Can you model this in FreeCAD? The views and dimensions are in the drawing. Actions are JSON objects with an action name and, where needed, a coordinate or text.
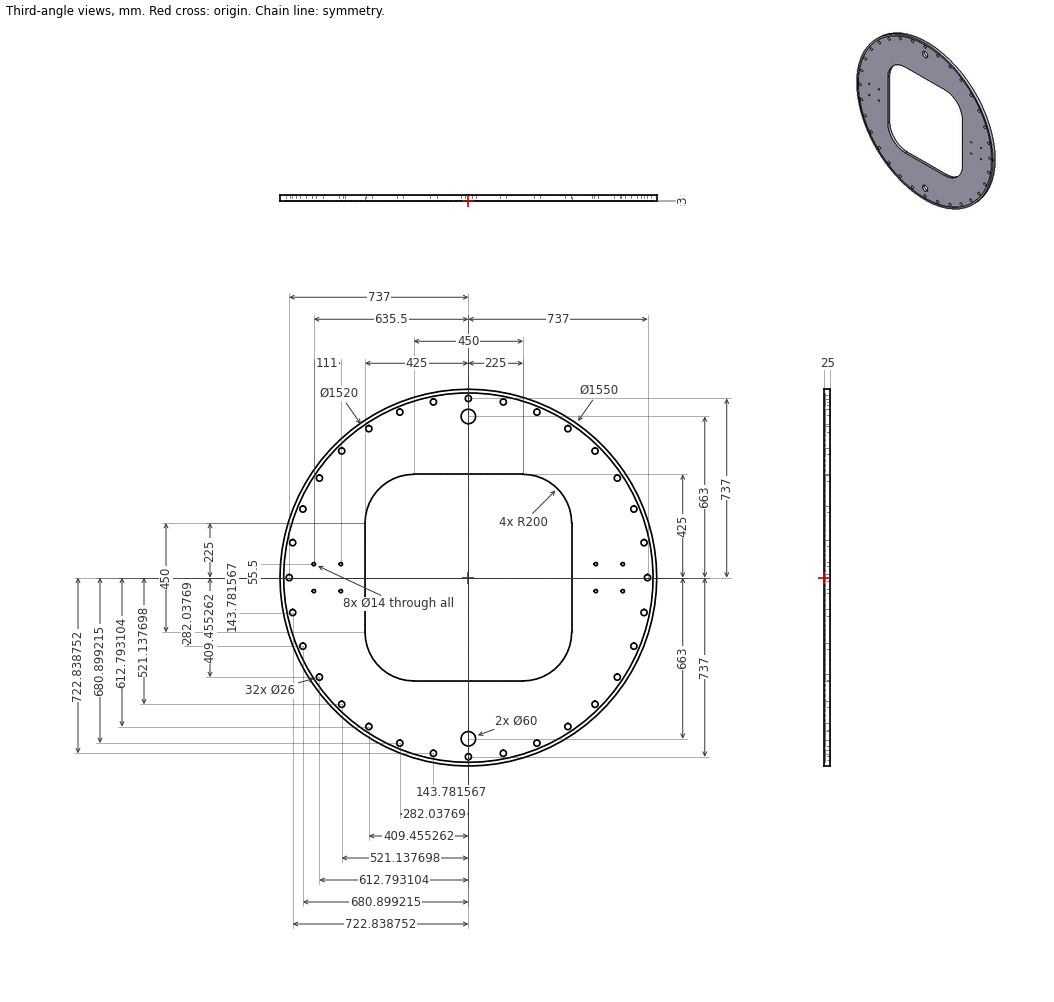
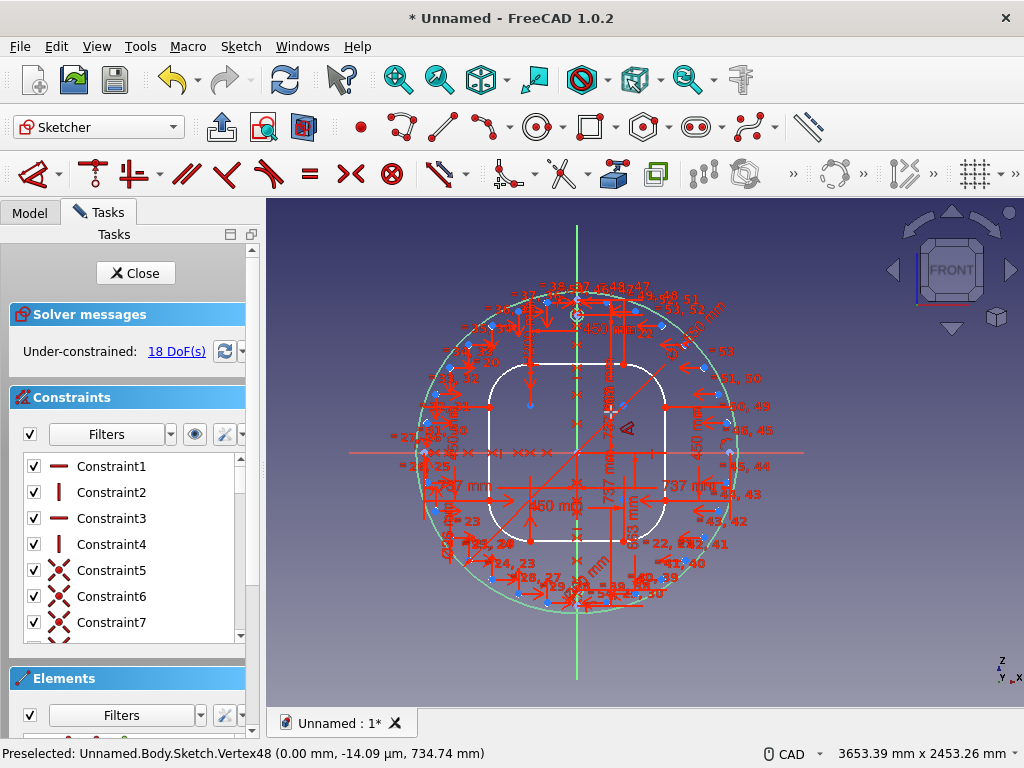
{"action": "left_click", "coordinate": [624, 364]}
{"action": "left_click", "coordinate": [617, 282]}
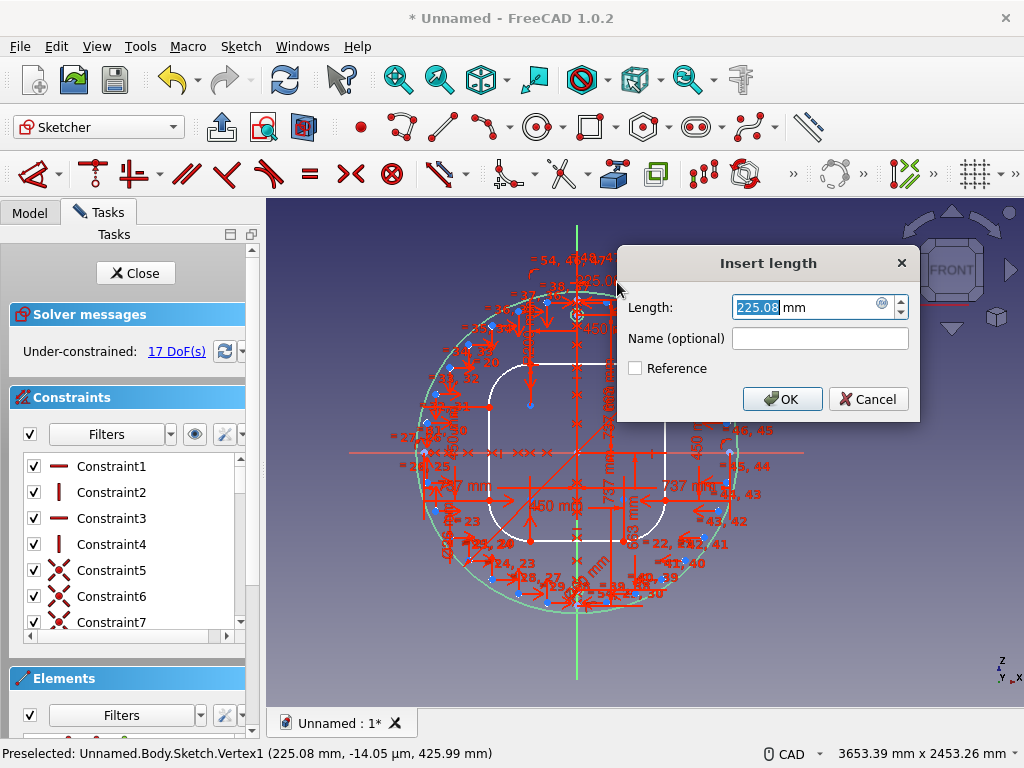
{"action": "type", "text": "225"}
{"action": "key", "text": "Return"}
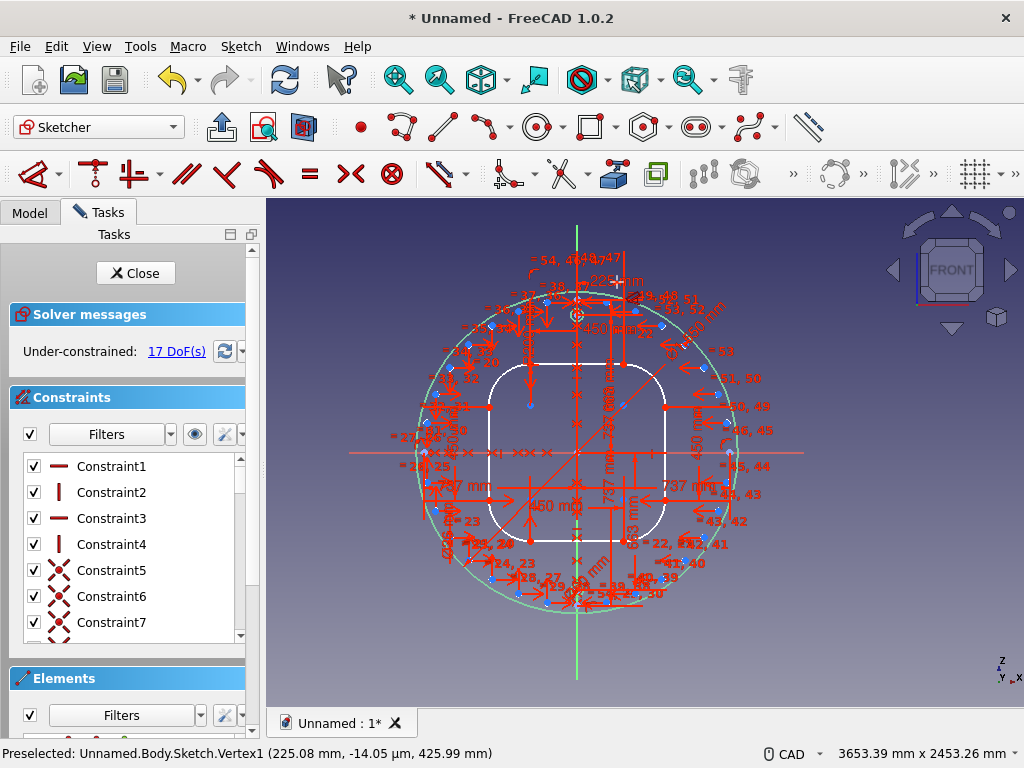
{"action": "left_click", "coordinate": [624, 364]}
{"action": "left_click", "coordinate": [543, 439]}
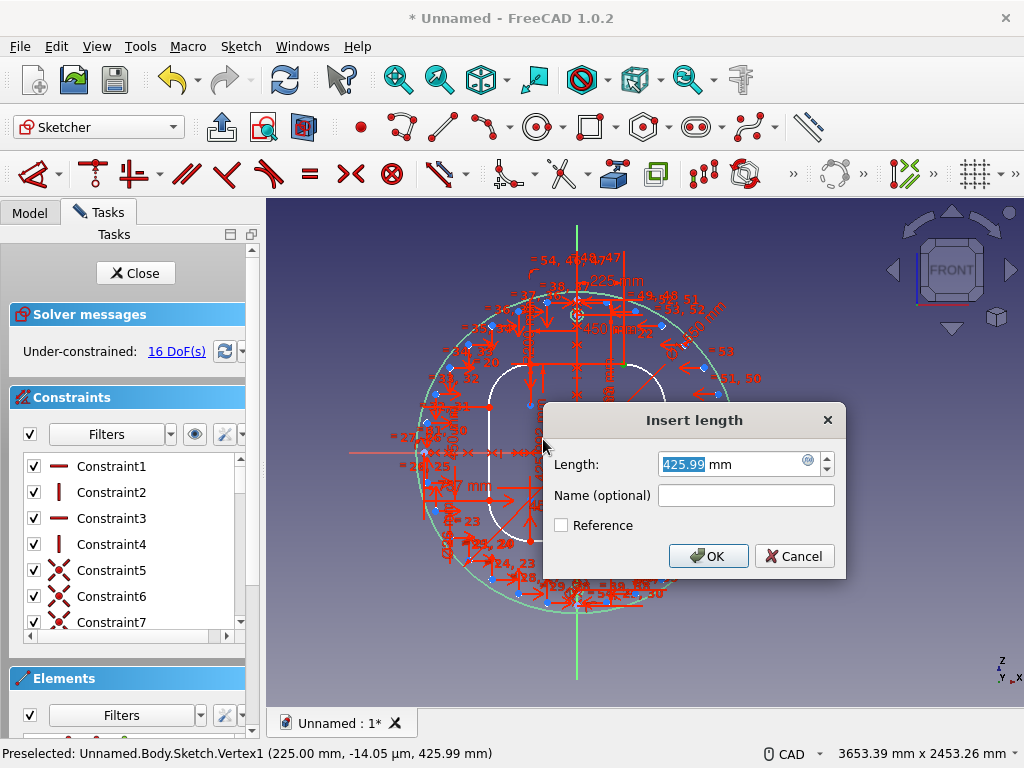
{"action": "type", "text": "425"}
{"action": "key", "text": "Return"}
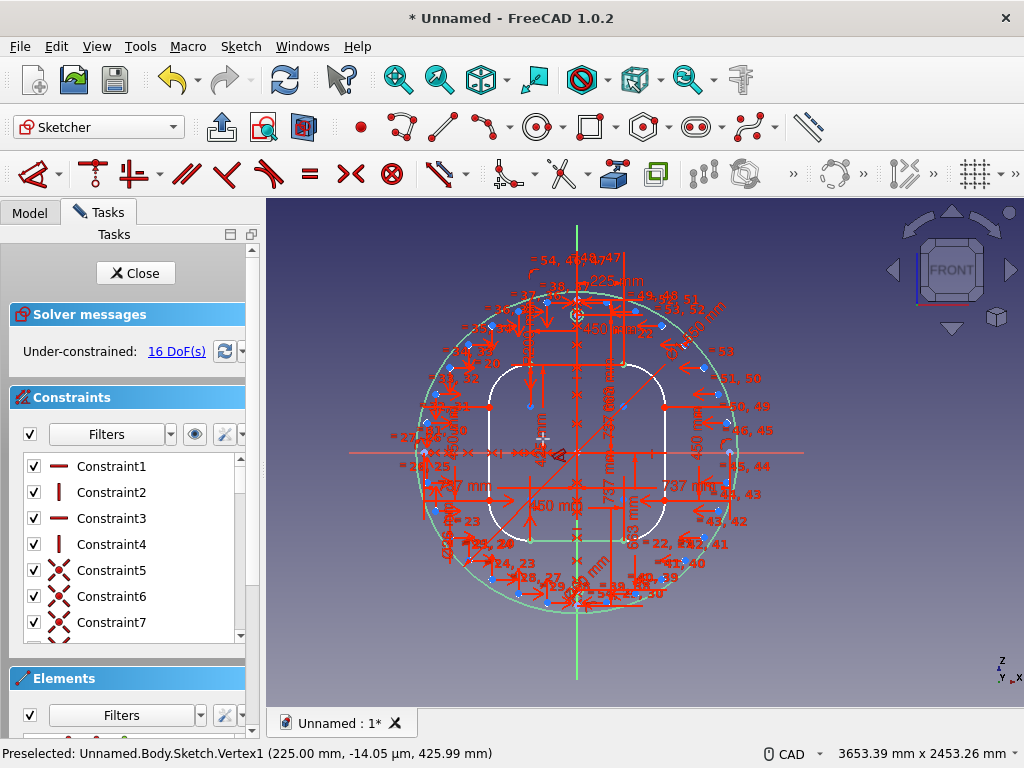
{"action": "left_click", "coordinate": [489, 407]}
{"action": "left_click", "coordinate": [533, 559]}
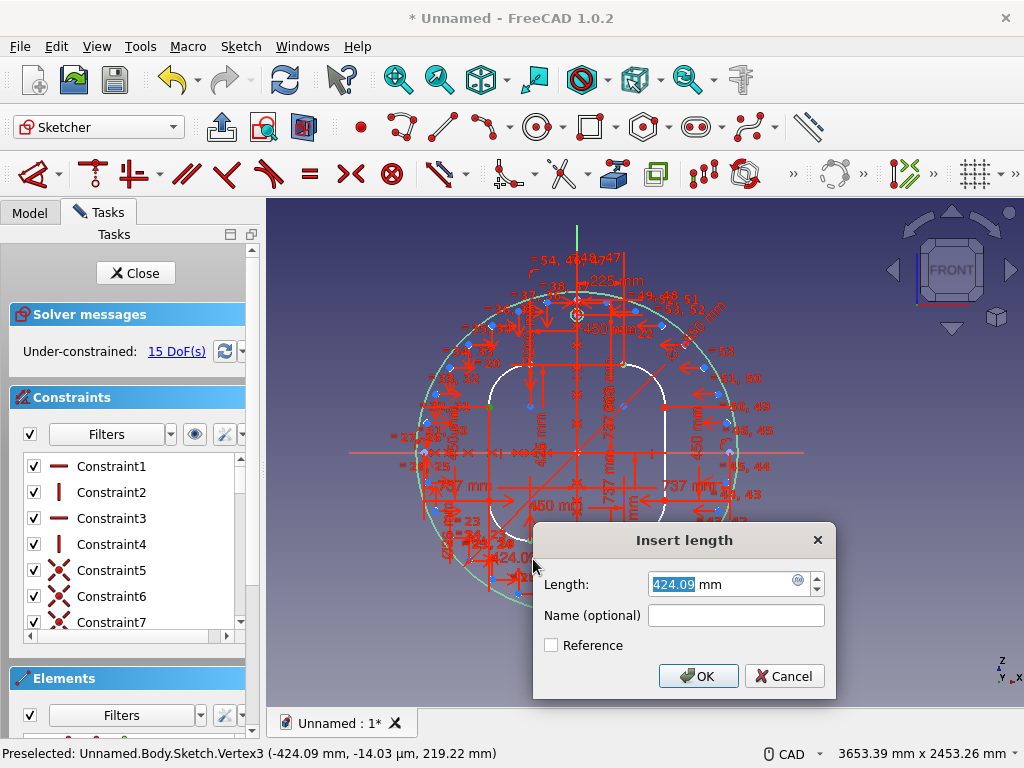
{"action": "type", "text": "425"}
{"action": "key", "text": "Return"}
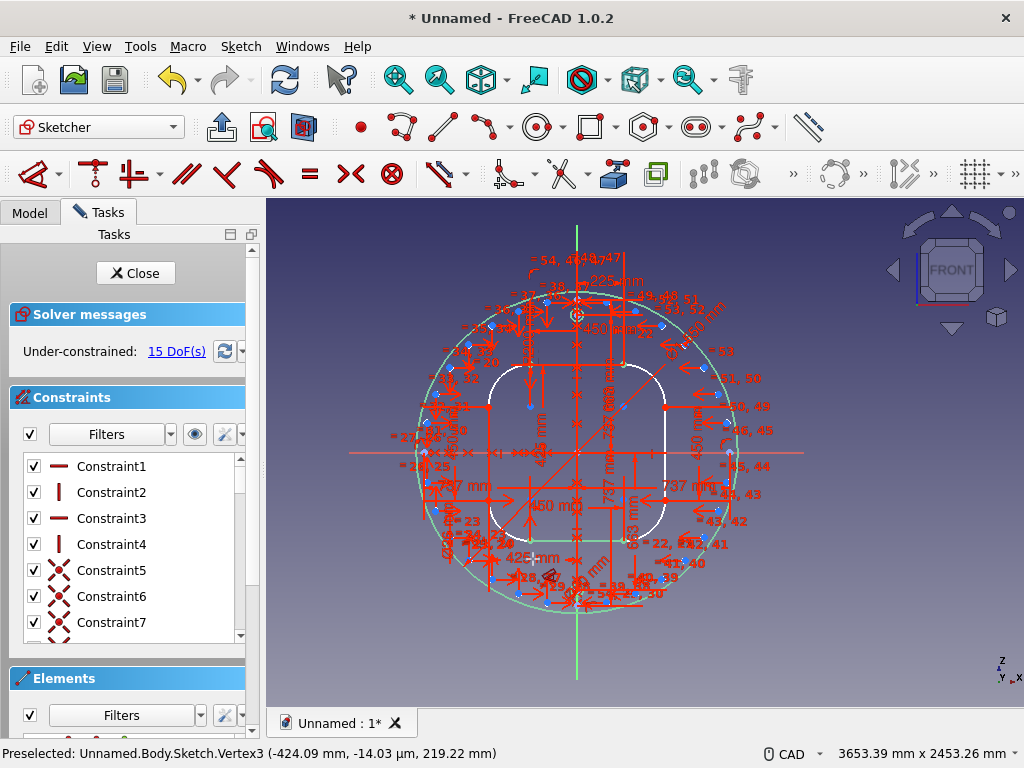
{"action": "left_click", "coordinate": [489, 407]}
{"action": "left_click", "coordinate": [383, 430]}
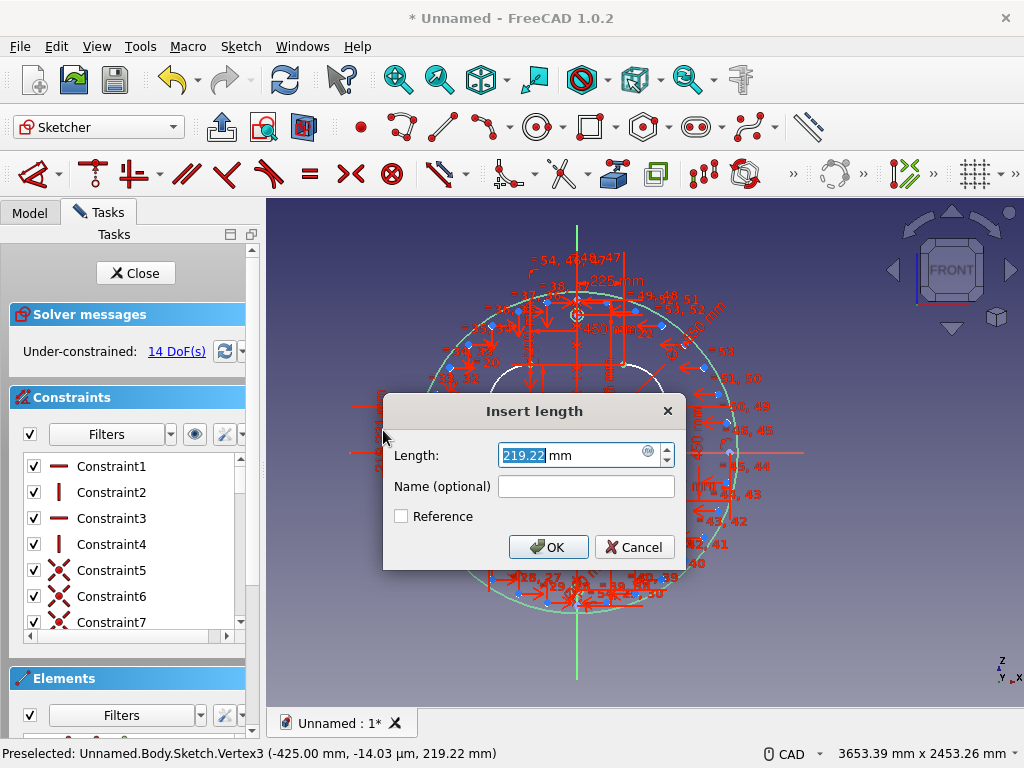
{"action": "type", "text": "225"}
{"action": "key", "text": "Return"}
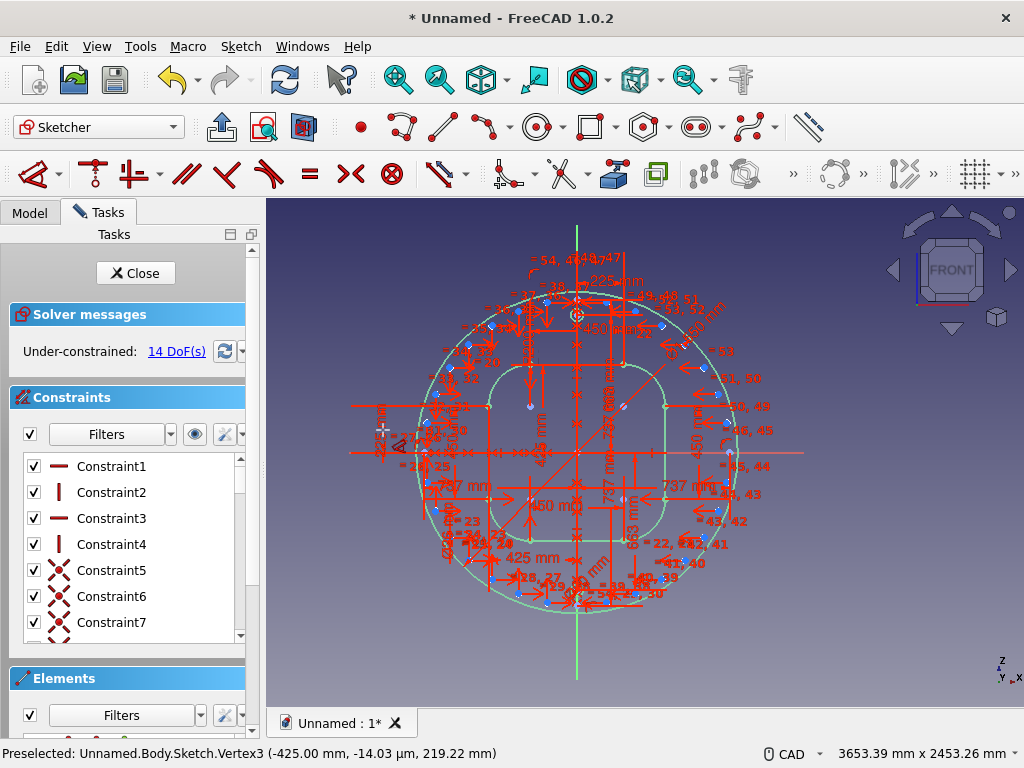
{"action": "left_click", "coordinate": [436, 511]}
{"action": "left_click", "coordinate": [378, 482]}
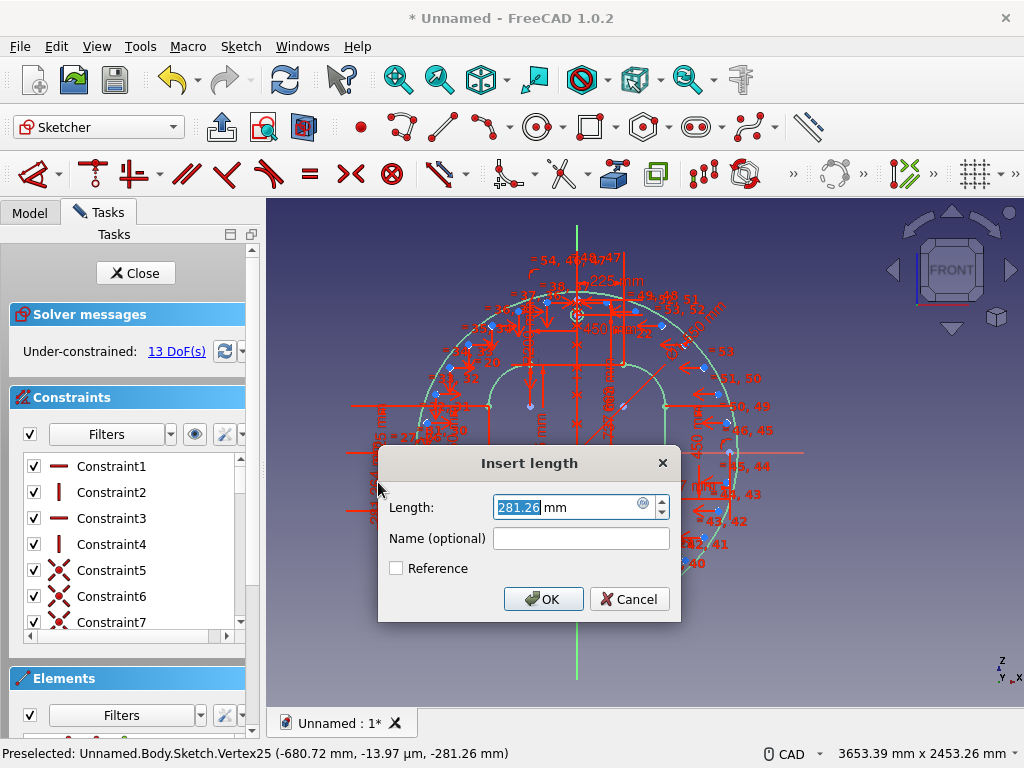
{"action": "type", "text": "282.03769"}
{"action": "key", "text": "Return"}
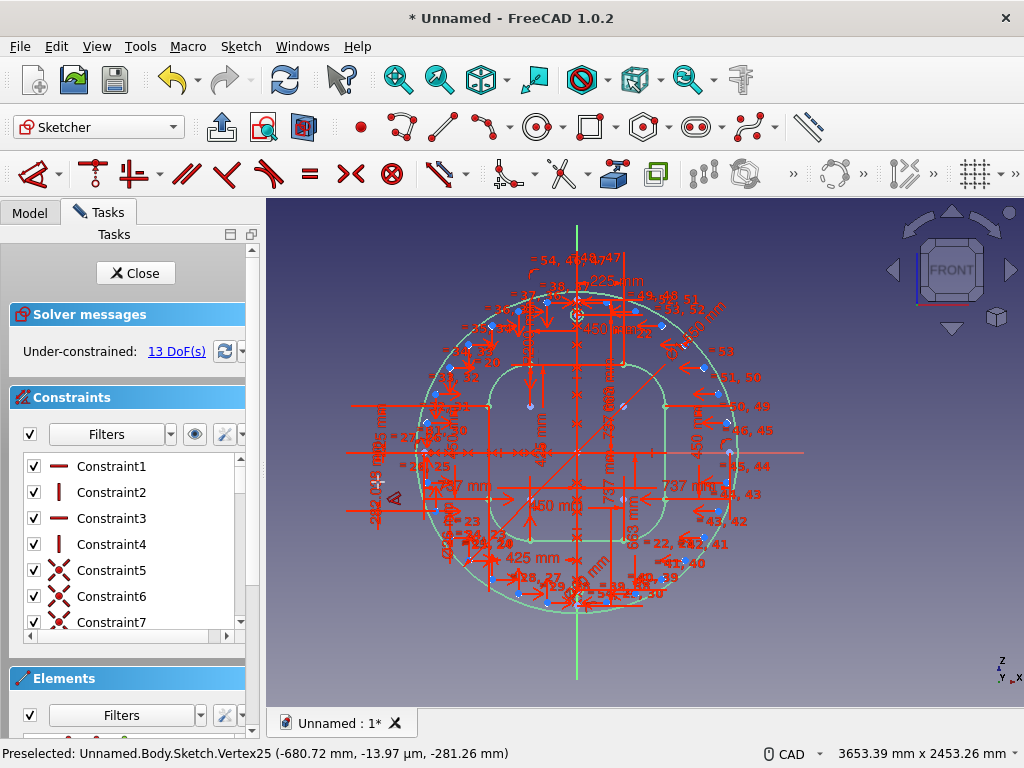
{"action": "left_click", "coordinate": [519, 594]}
{"action": "left_click", "coordinate": [548, 628]}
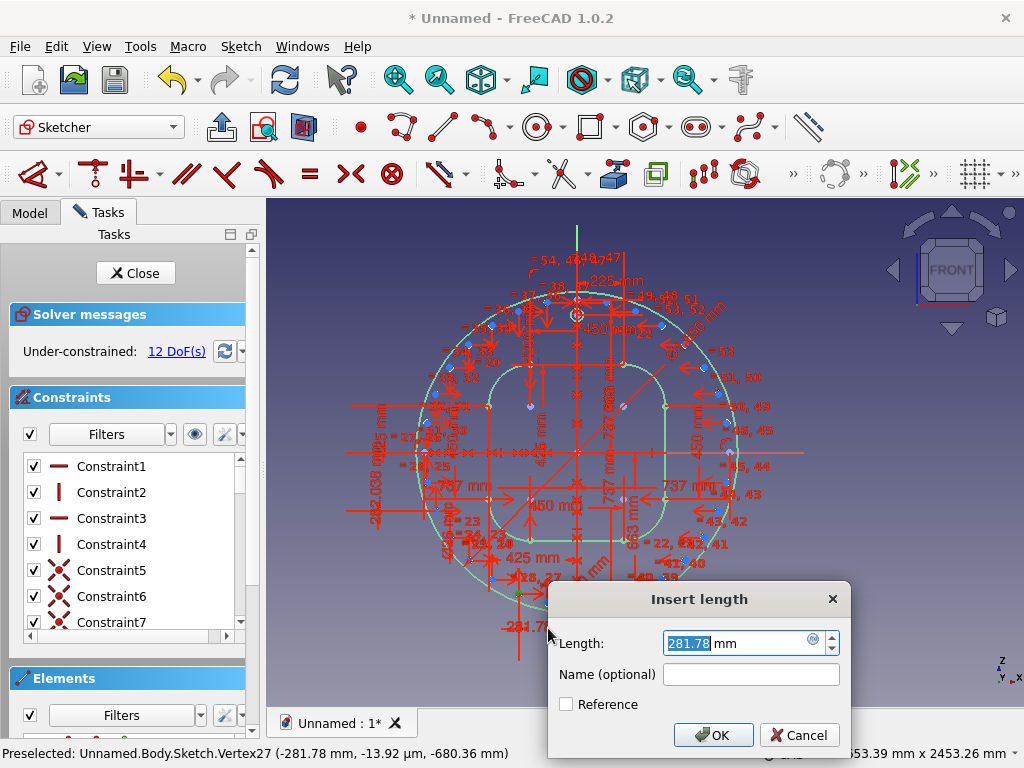
{"action": "type", "text": "282.03769"}
{"action": "key", "text": "Return"}